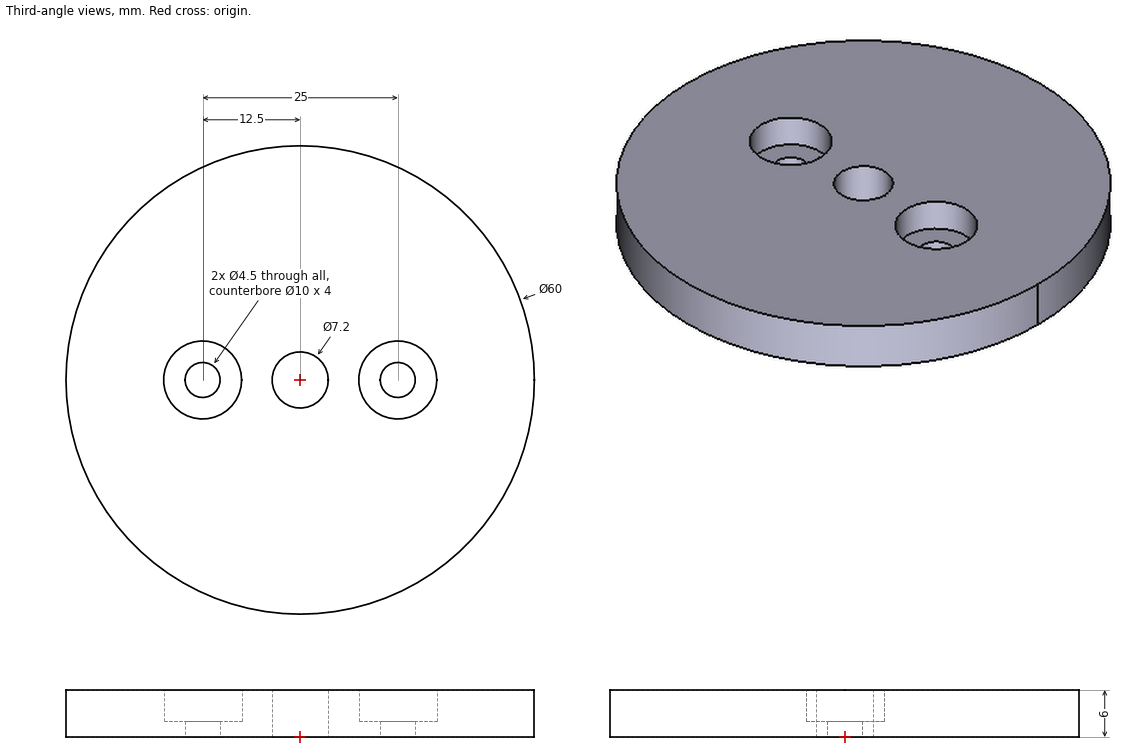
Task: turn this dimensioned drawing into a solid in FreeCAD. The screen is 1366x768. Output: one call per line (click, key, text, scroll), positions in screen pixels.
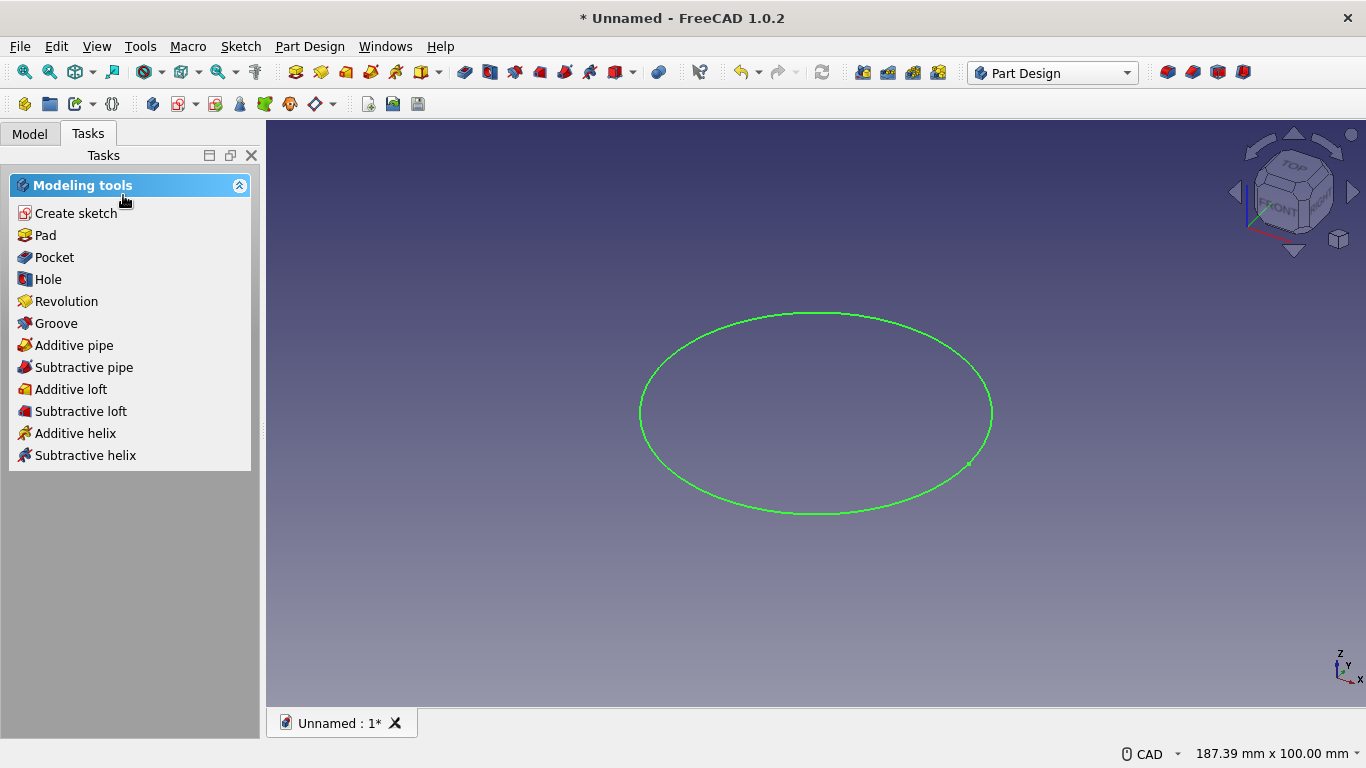
click(296, 72)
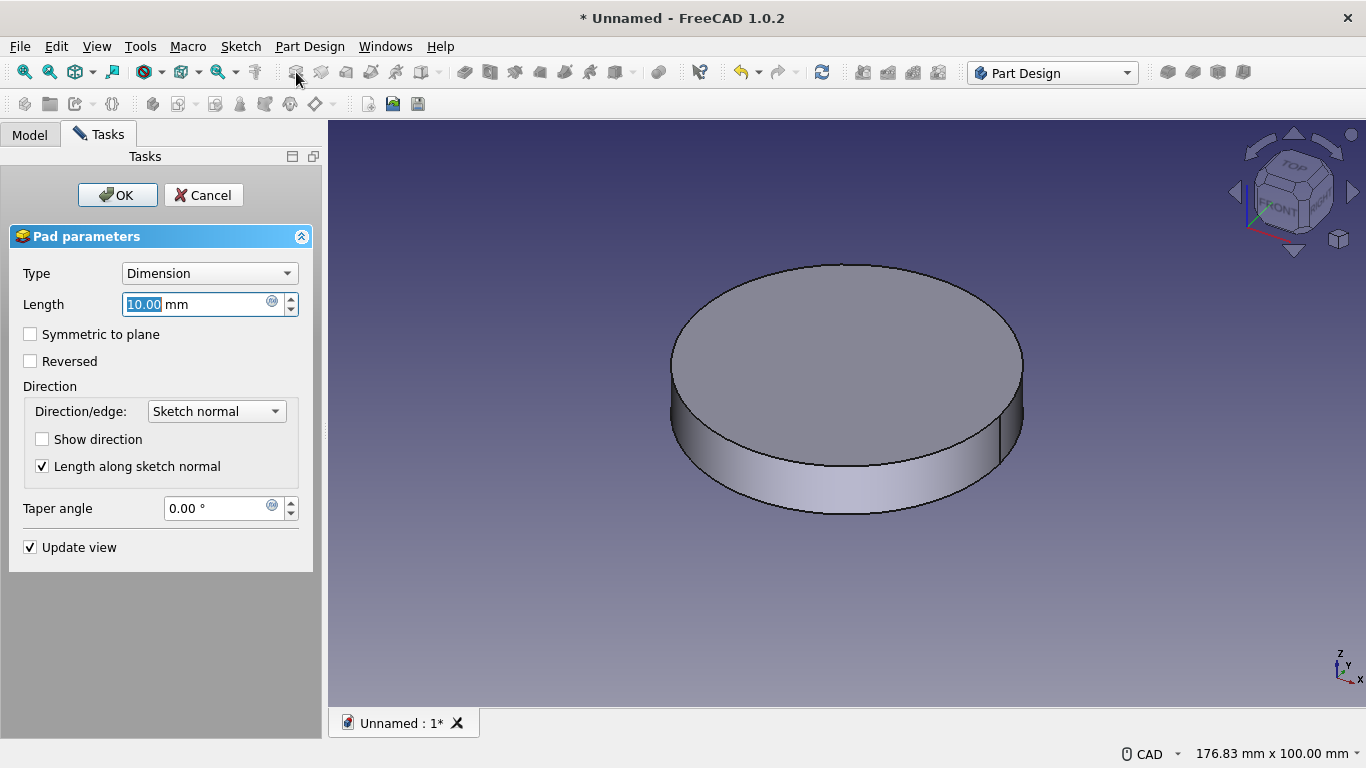
text(6)
key(Tab)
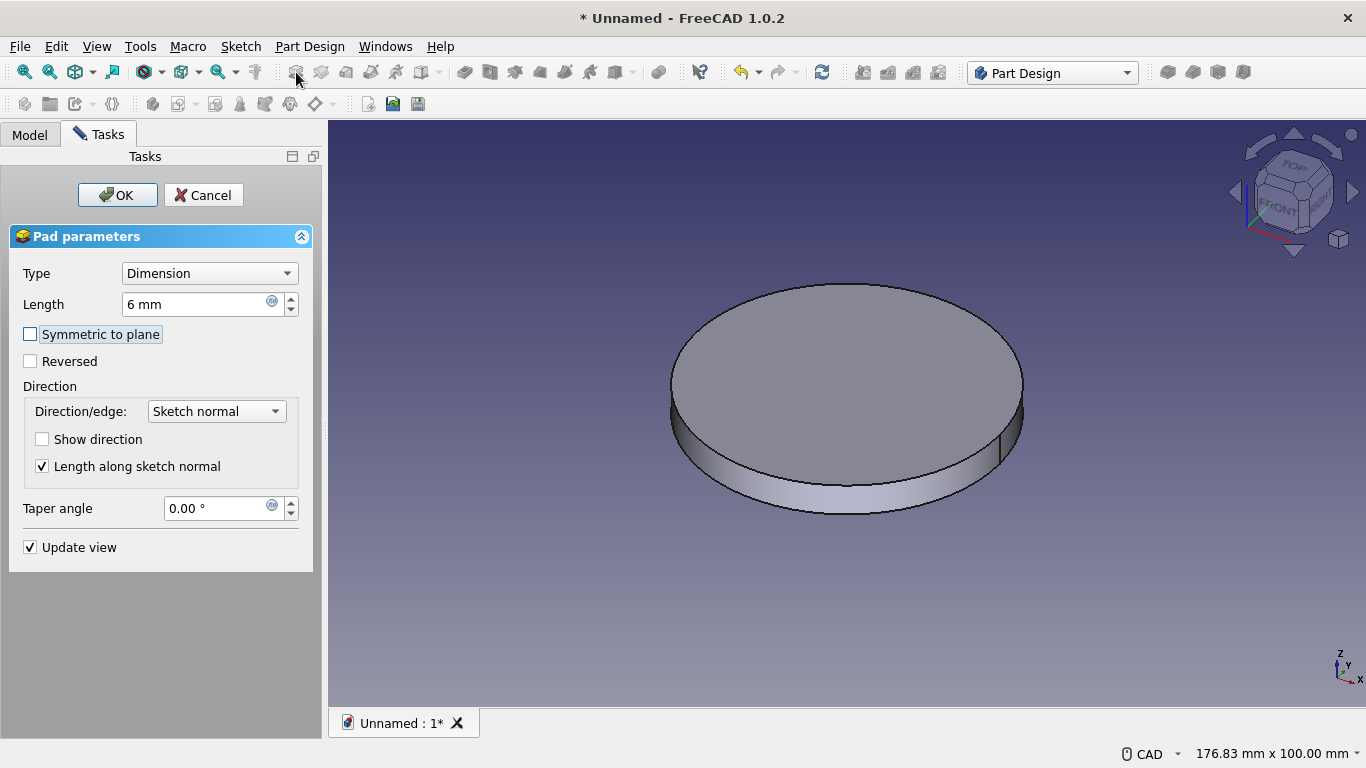
click(118, 195)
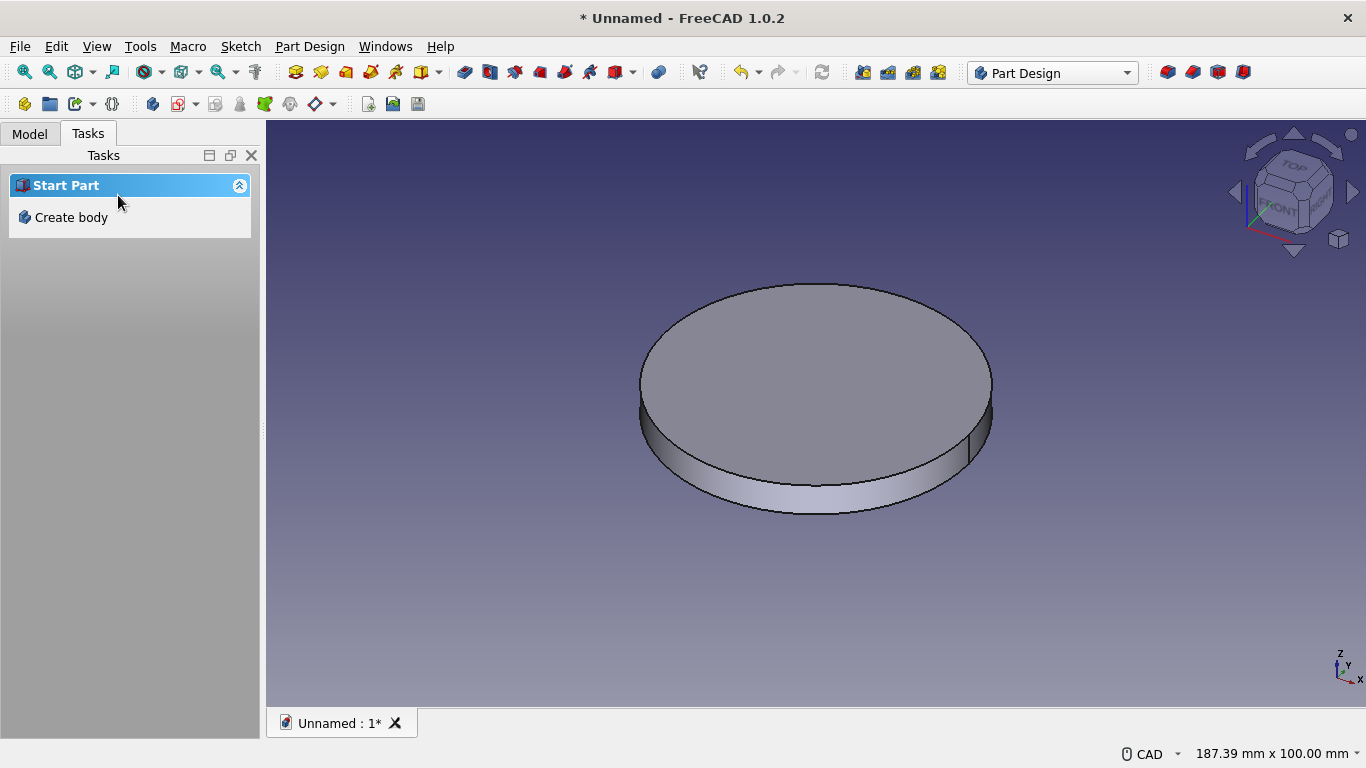
click(816, 384)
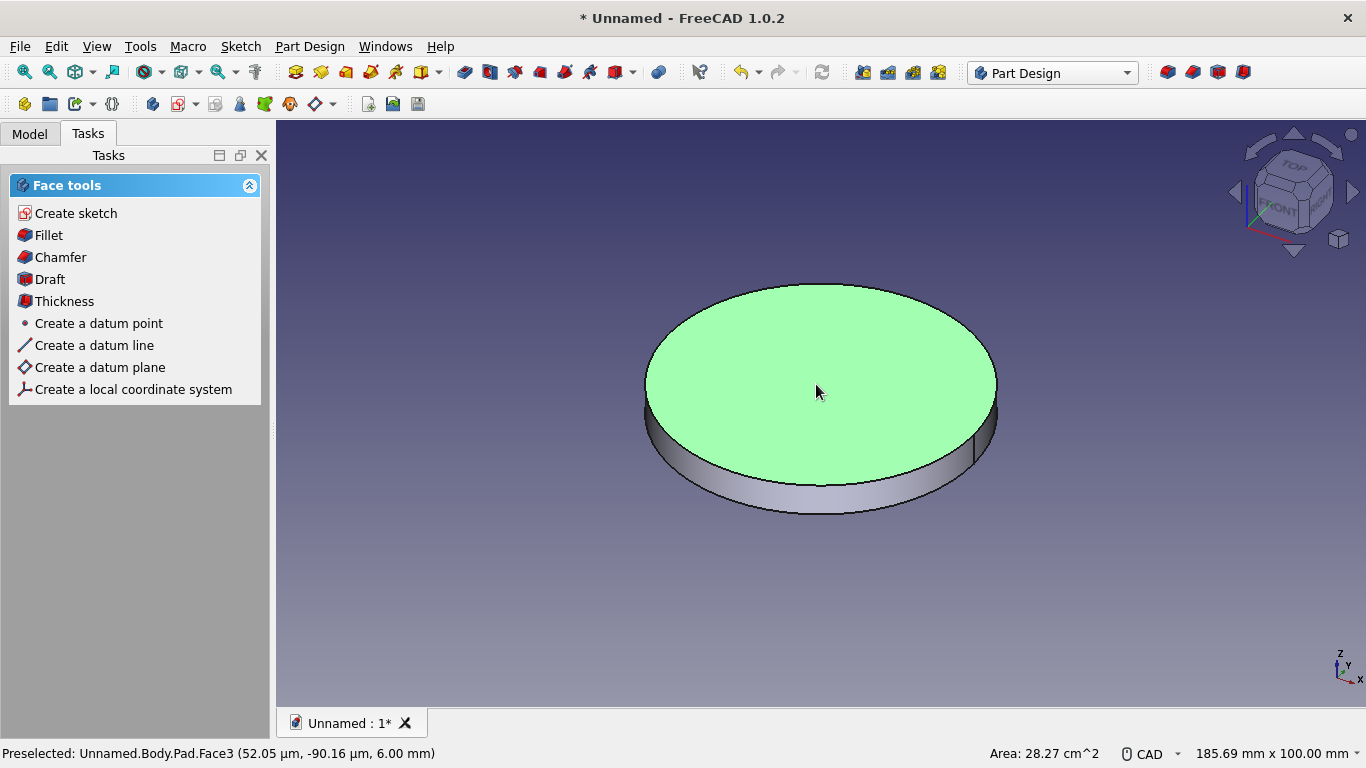
click(178, 104)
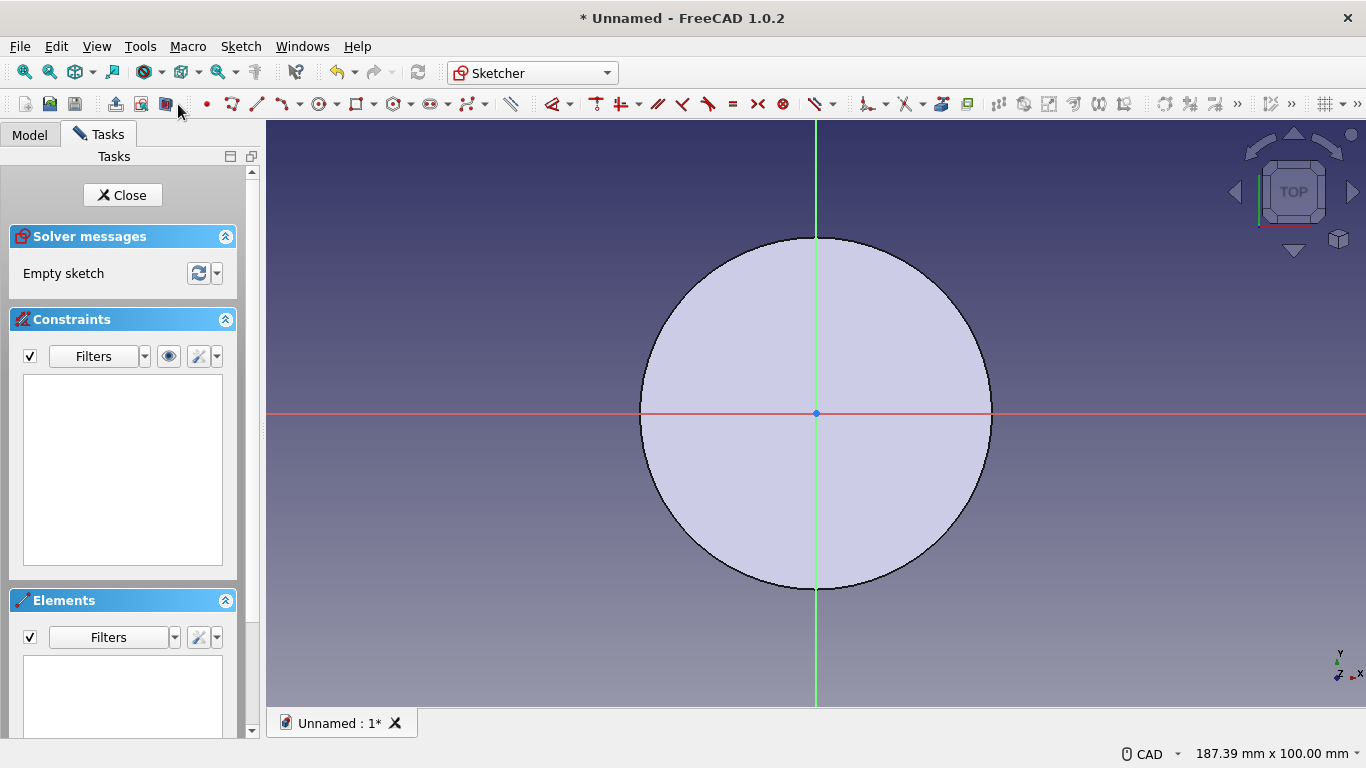
scroll(838, 414, up, 7)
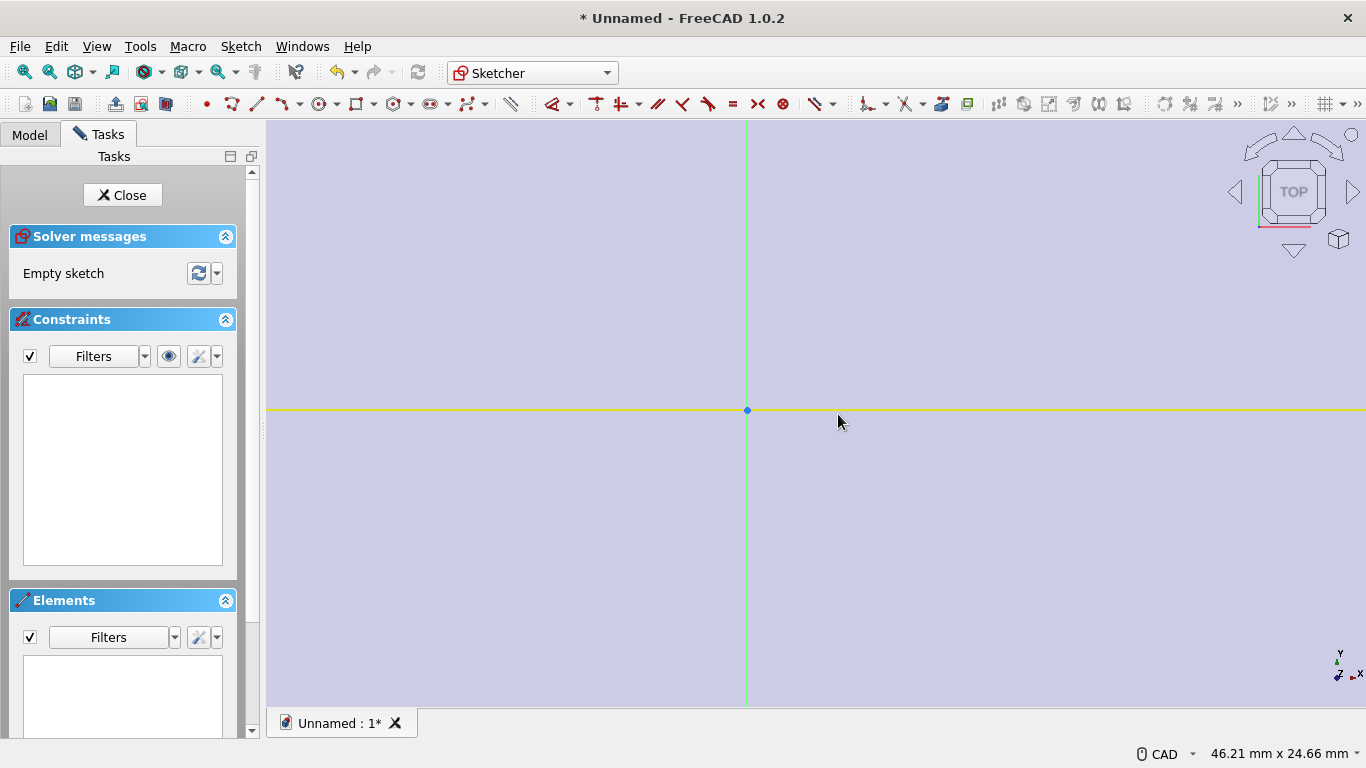
click(318, 104)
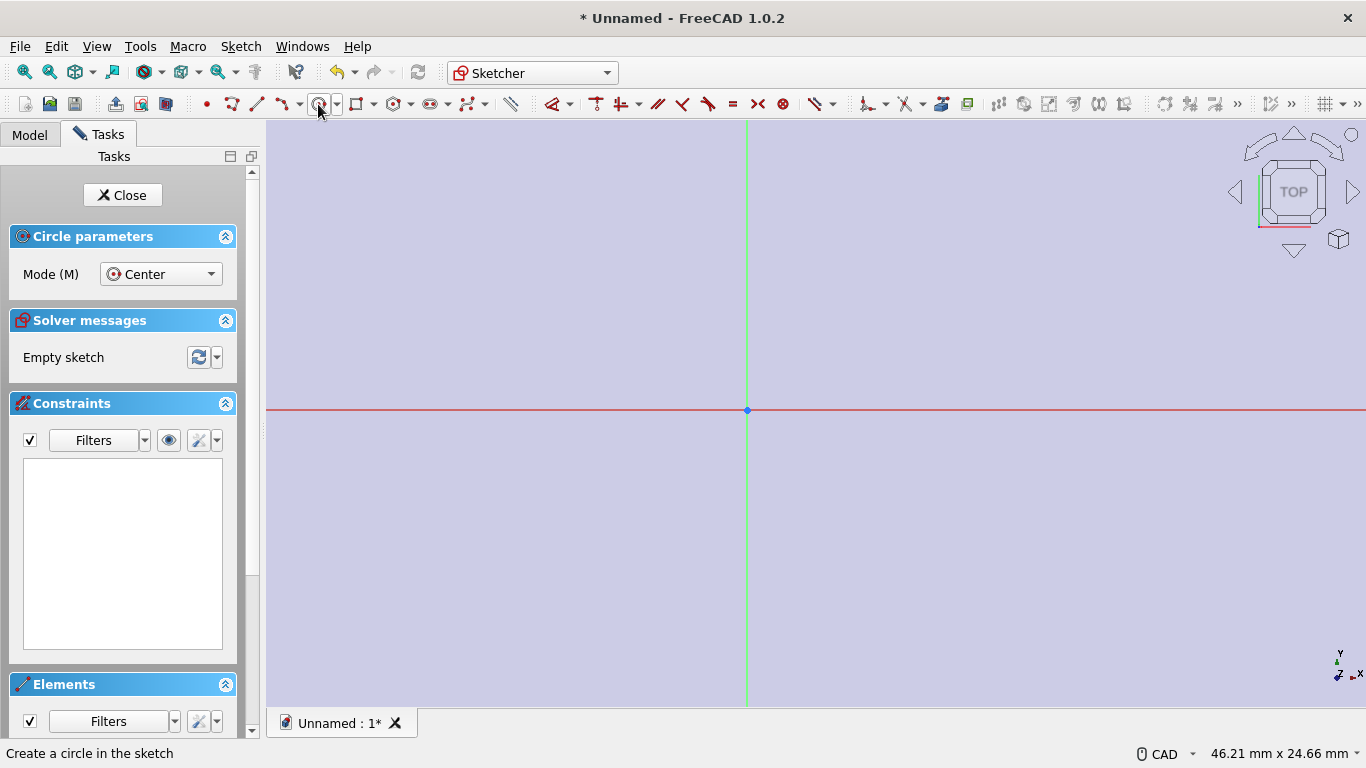
click(450, 410)
click(488, 373)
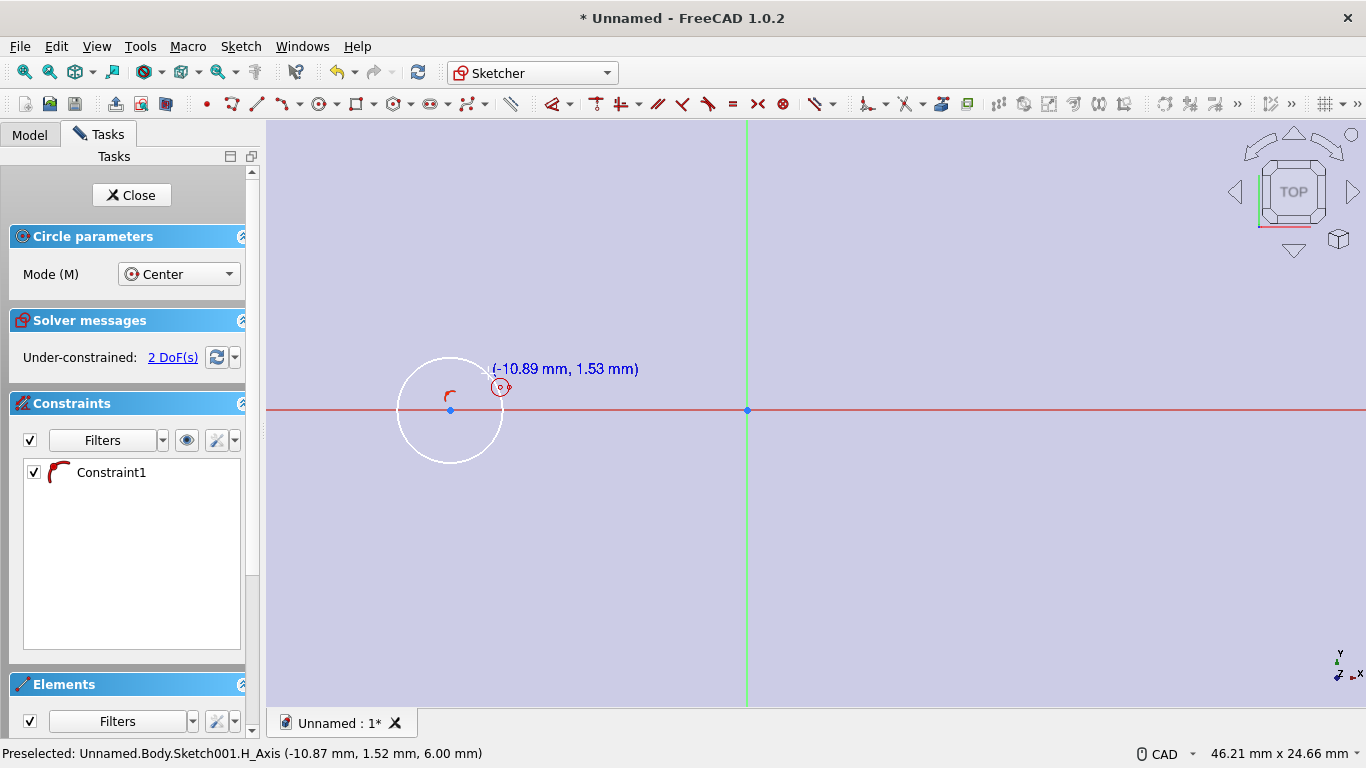
click(1045, 410)
click(1083, 373)
key(Escape)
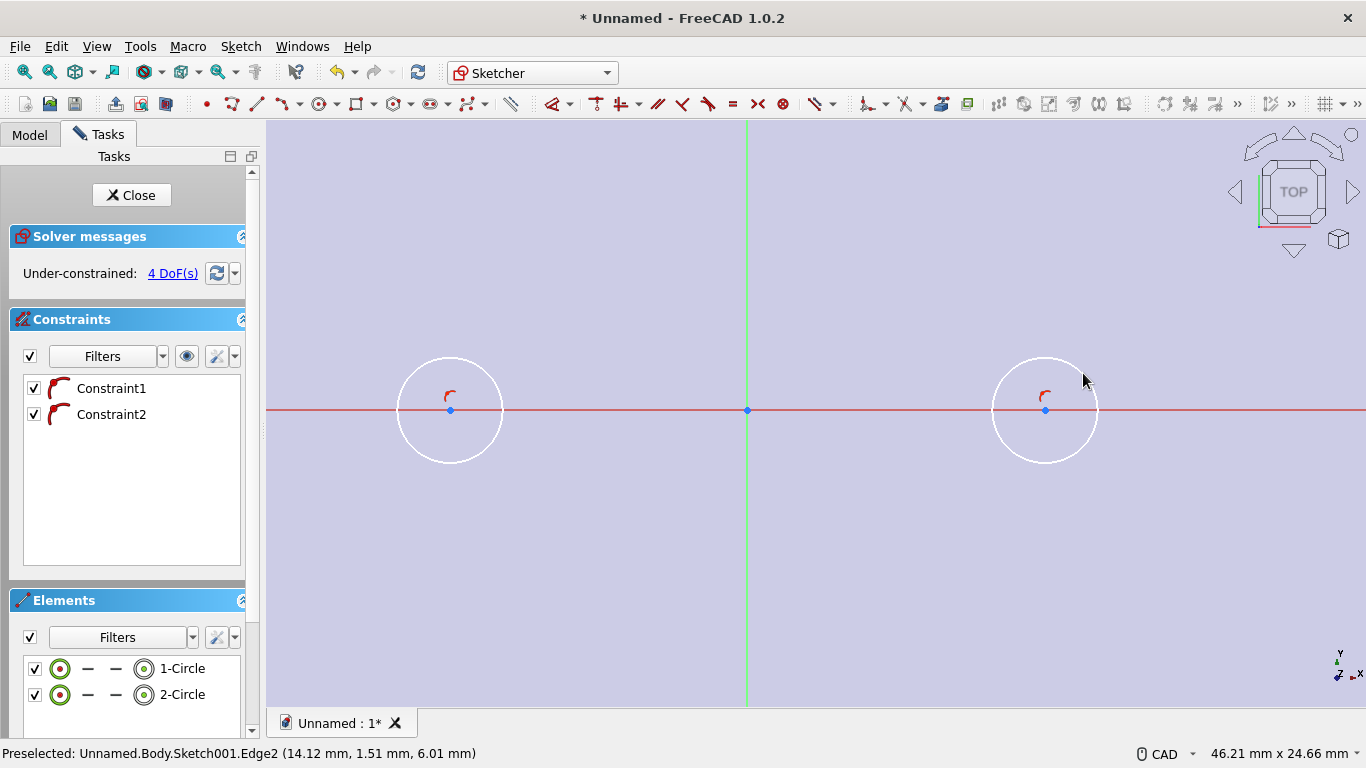
click(487, 373)